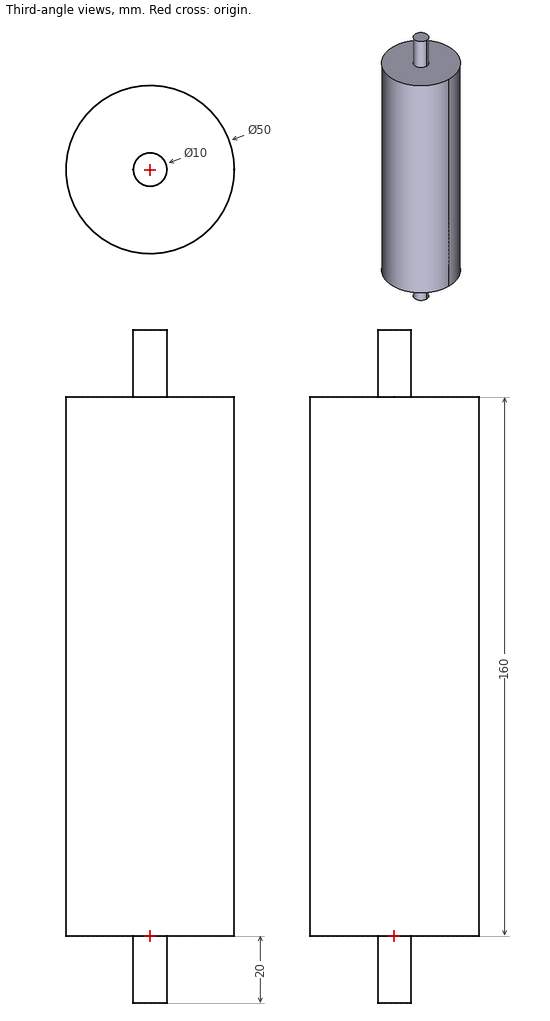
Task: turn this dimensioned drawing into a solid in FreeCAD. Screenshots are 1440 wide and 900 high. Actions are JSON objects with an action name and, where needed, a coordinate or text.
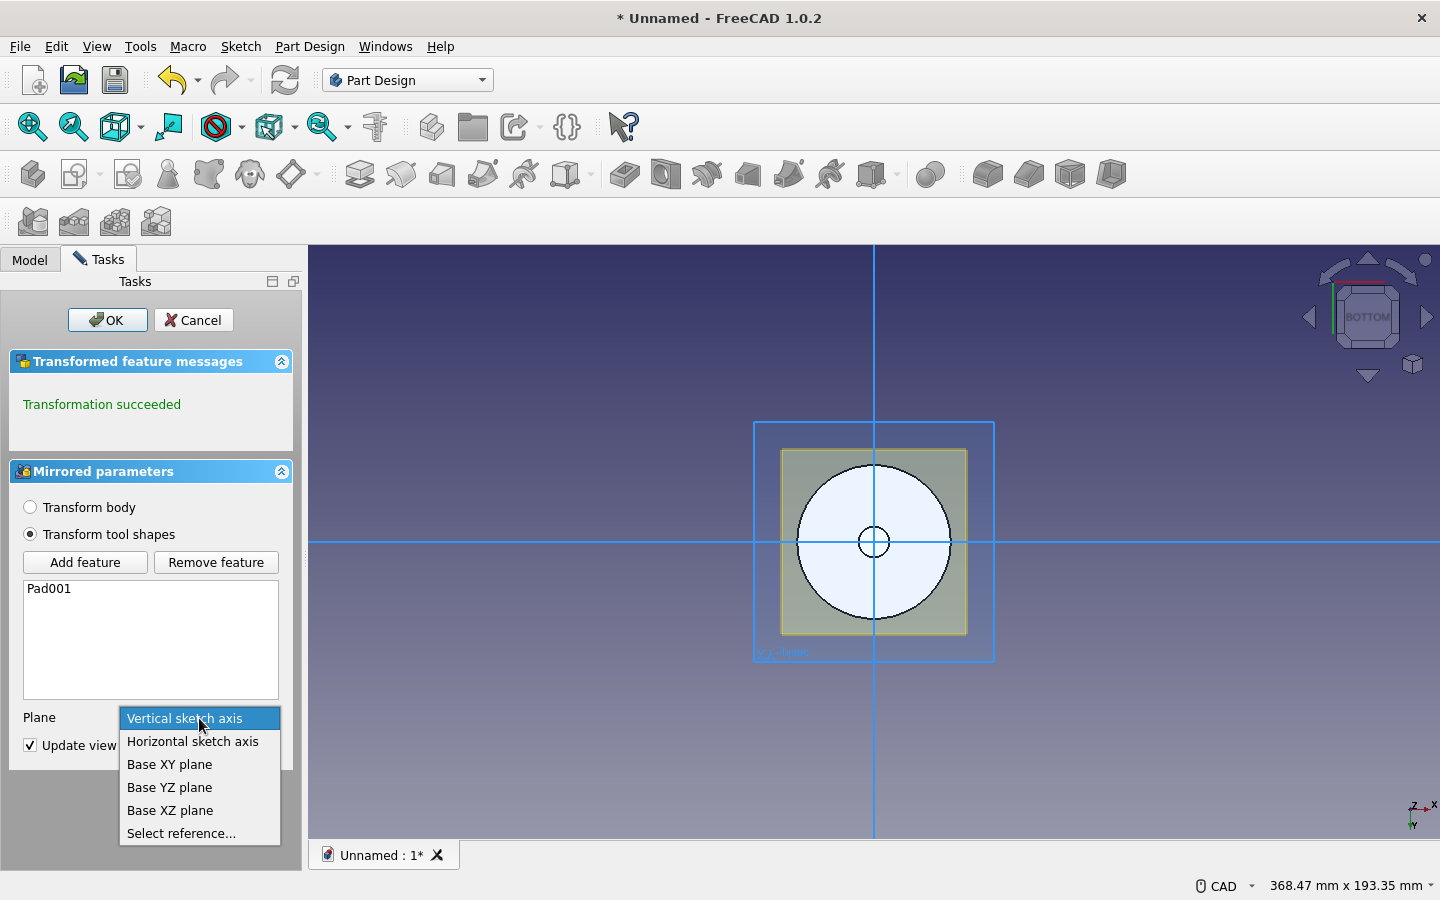
{"action": "left_click", "coordinate": [198, 834]}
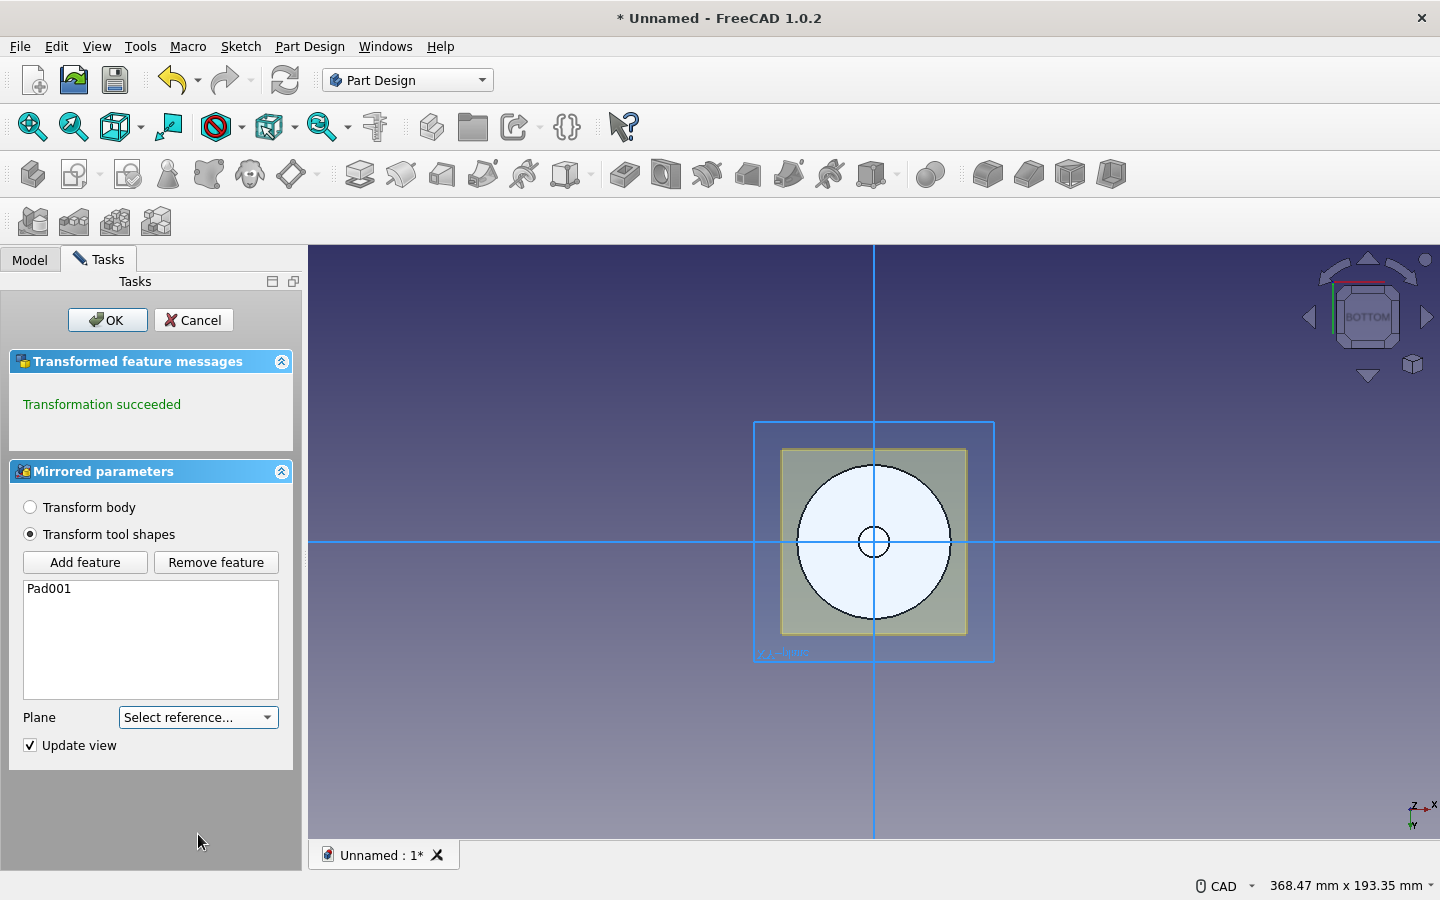
{"action": "left_click", "coordinate": [30, 259]}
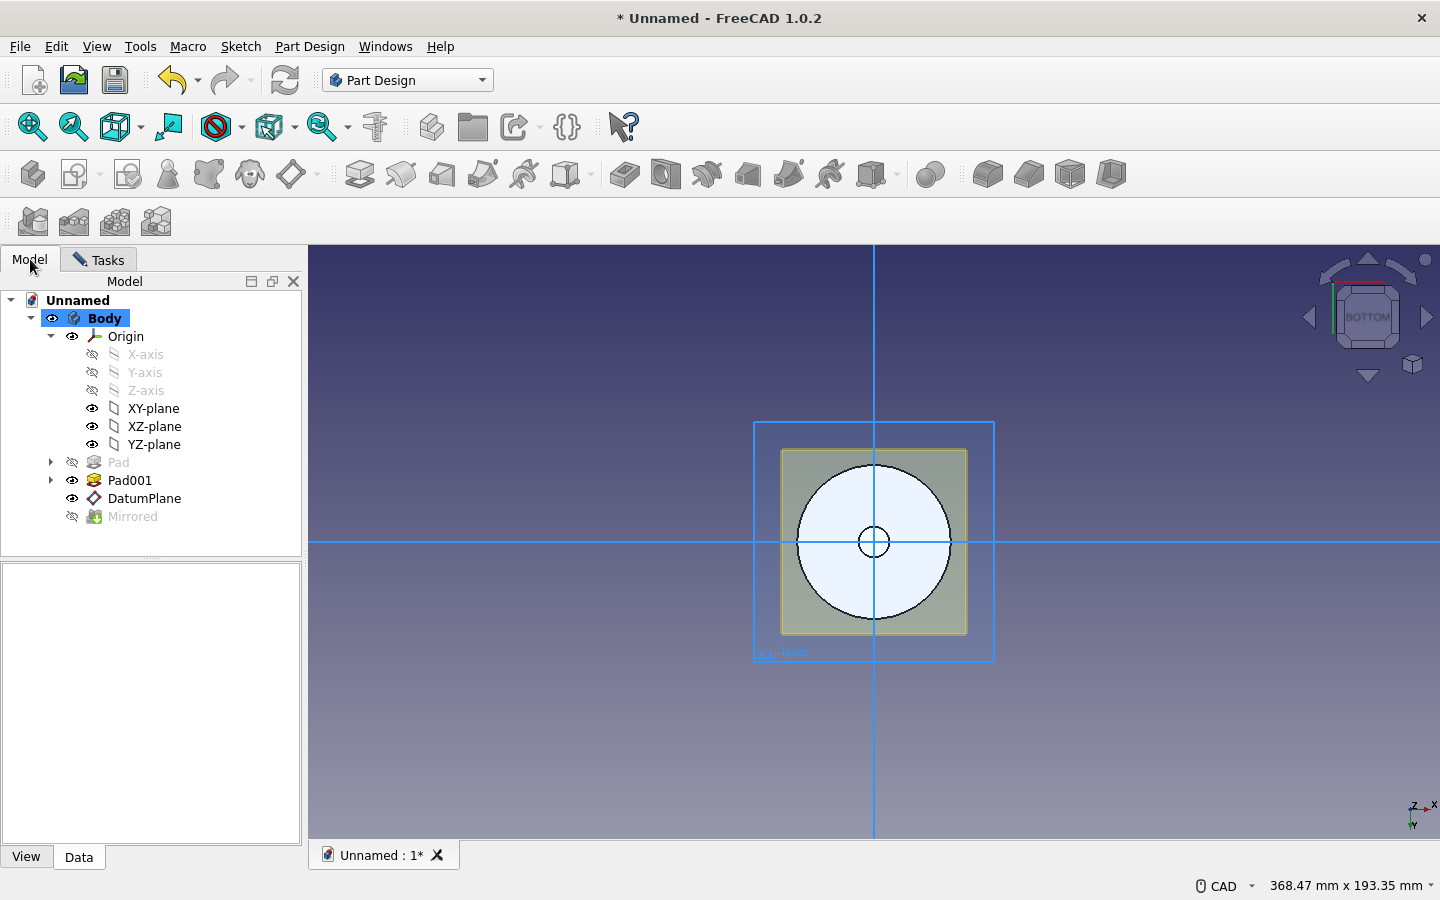
{"action": "left_click", "coordinate": [117, 498]}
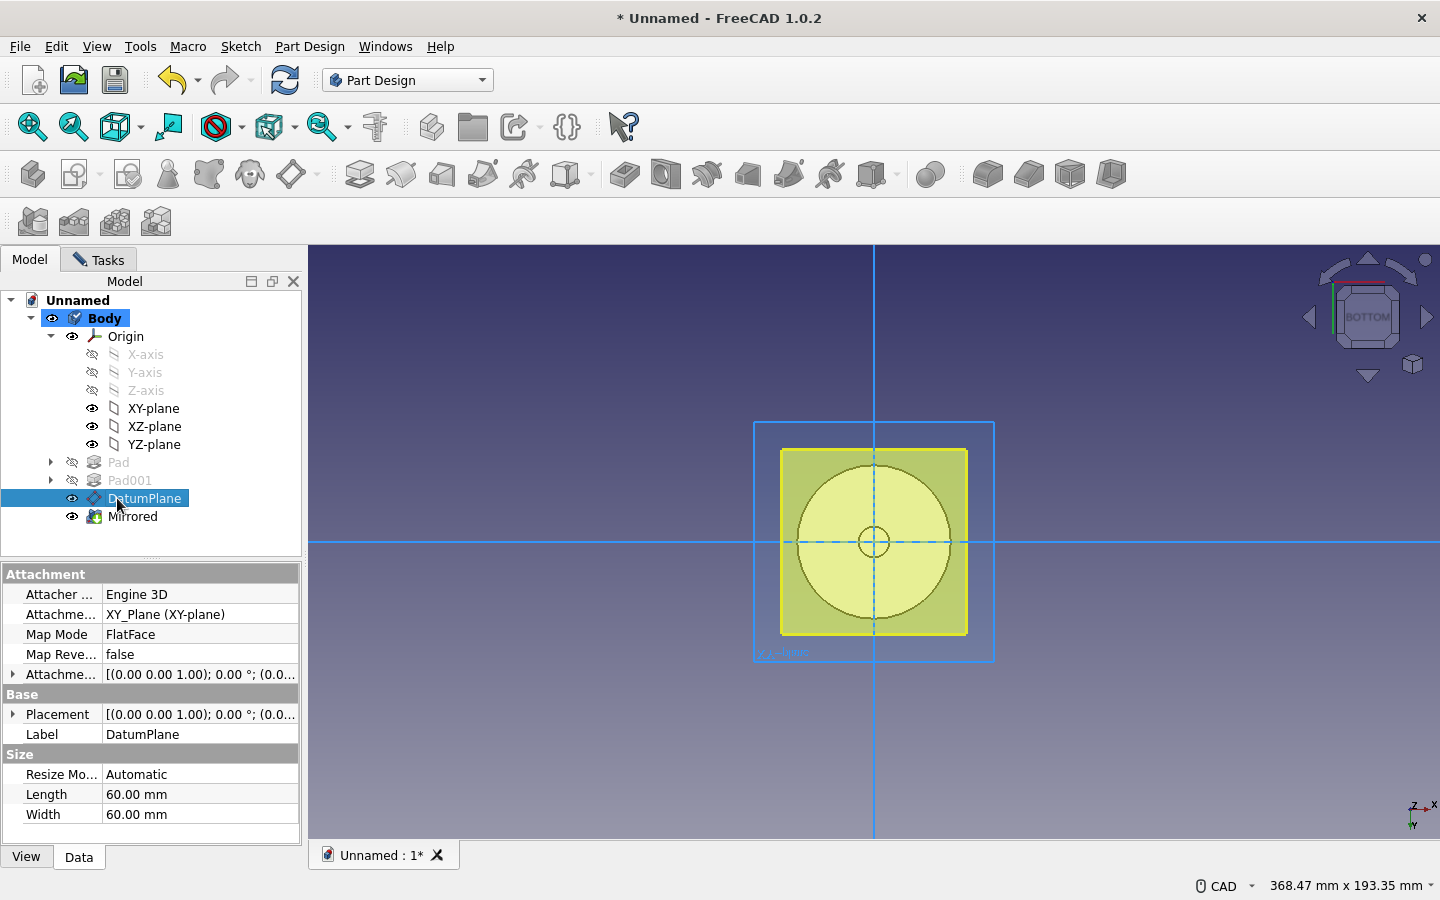
{"action": "left_click", "coordinate": [98, 259]}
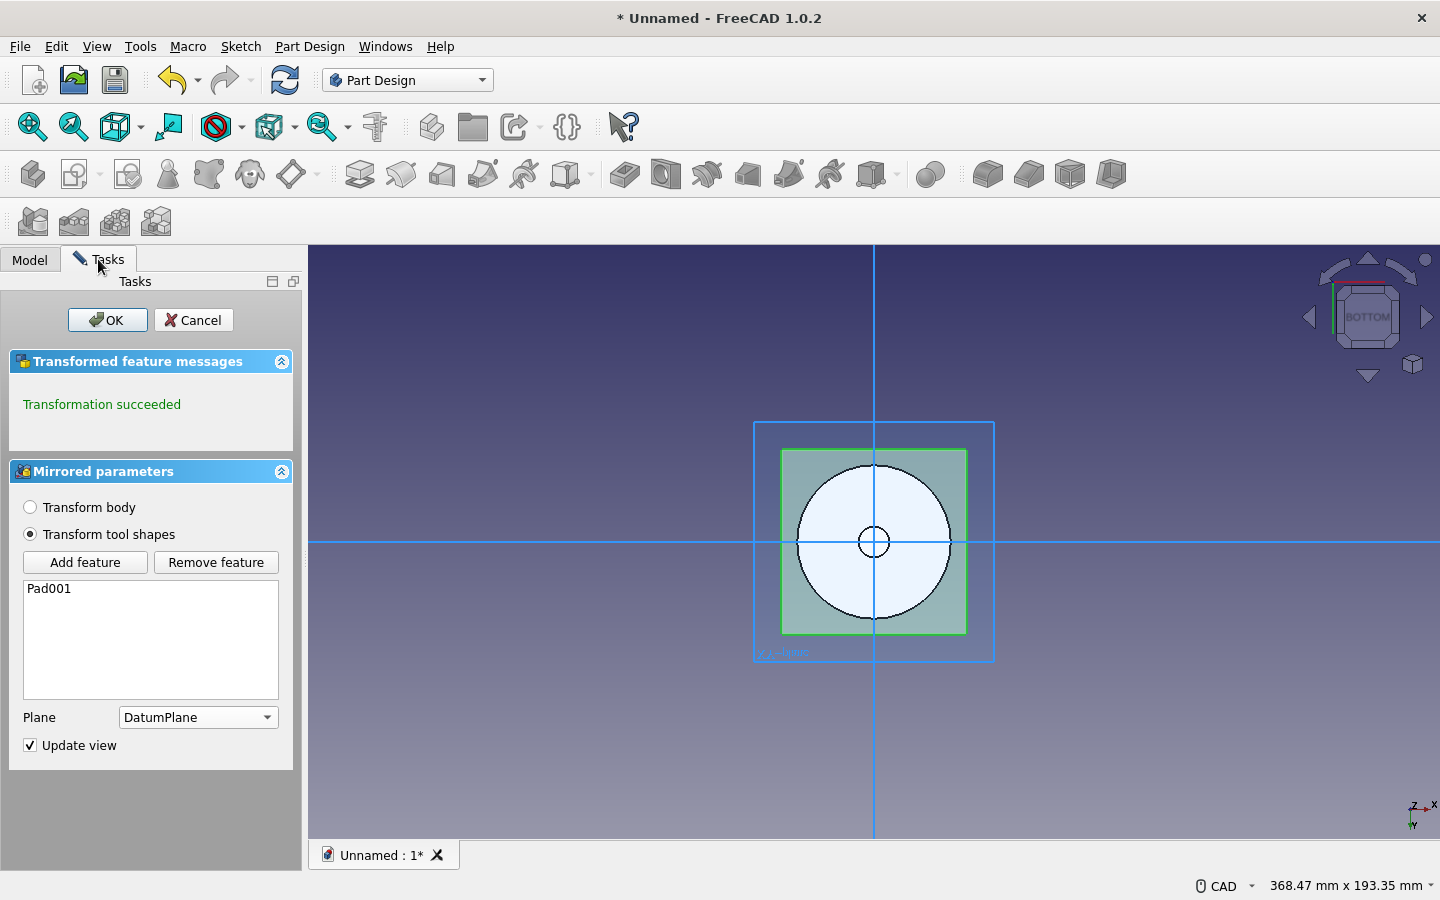
{"action": "left_click", "coordinate": [108, 320]}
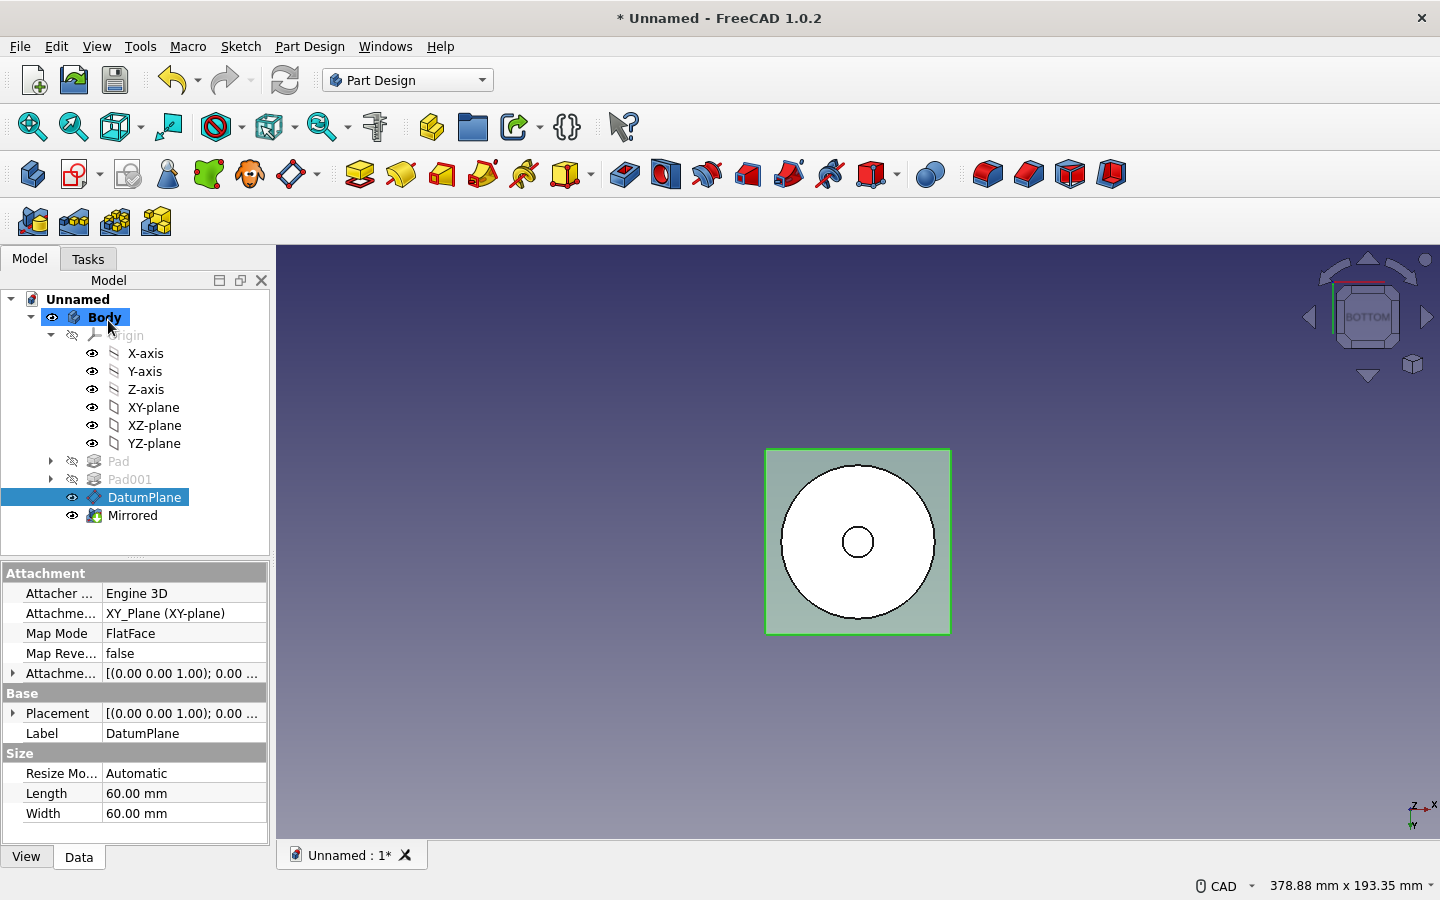
{"action": "left_click", "coordinate": [117, 497]}
{"action": "key", "text": "space"}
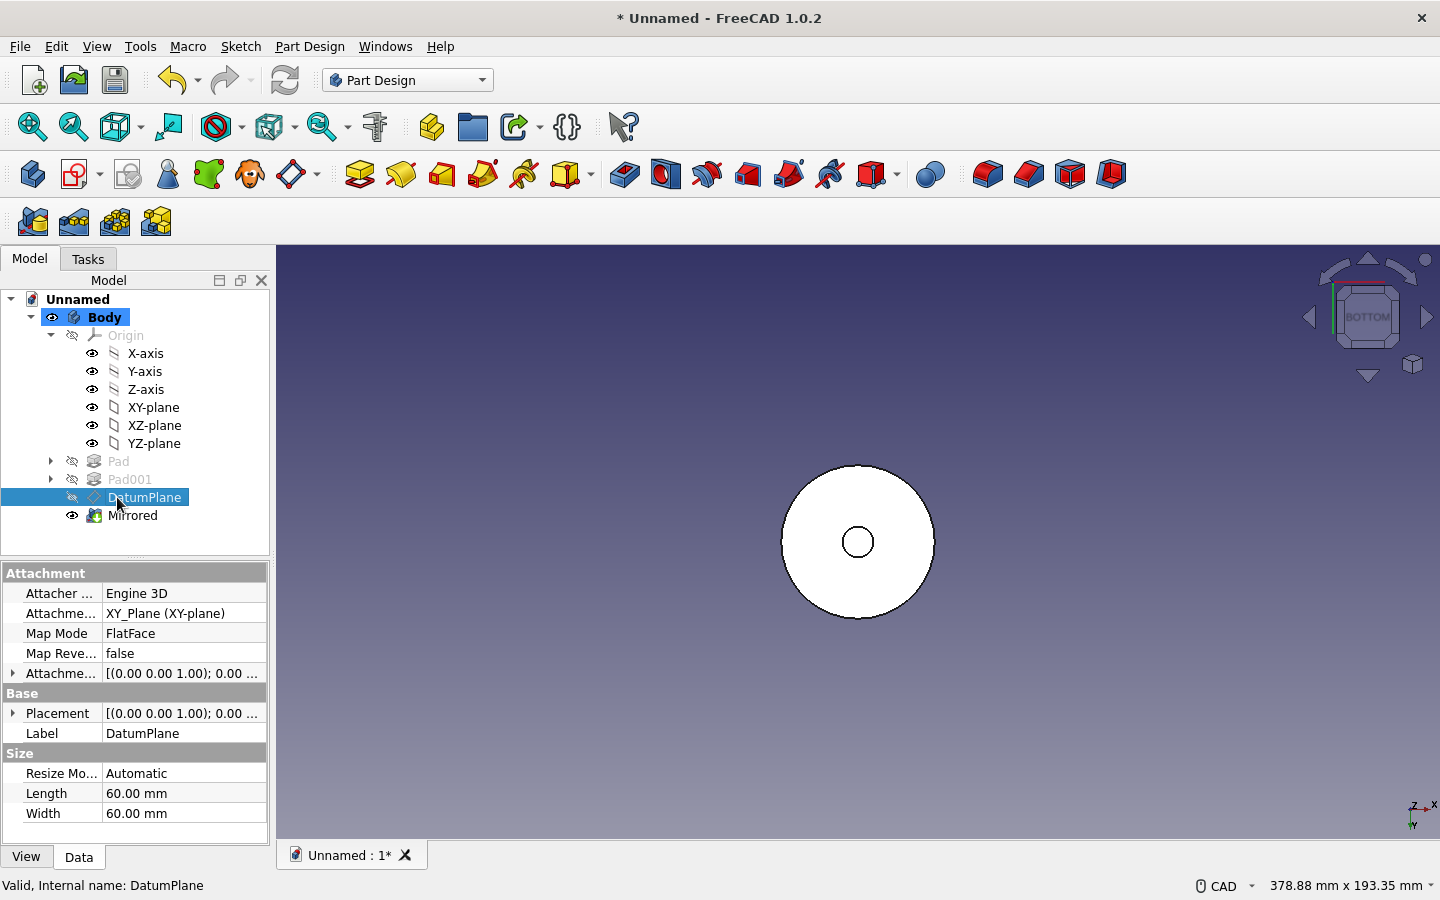
{"action": "key", "text": "0"}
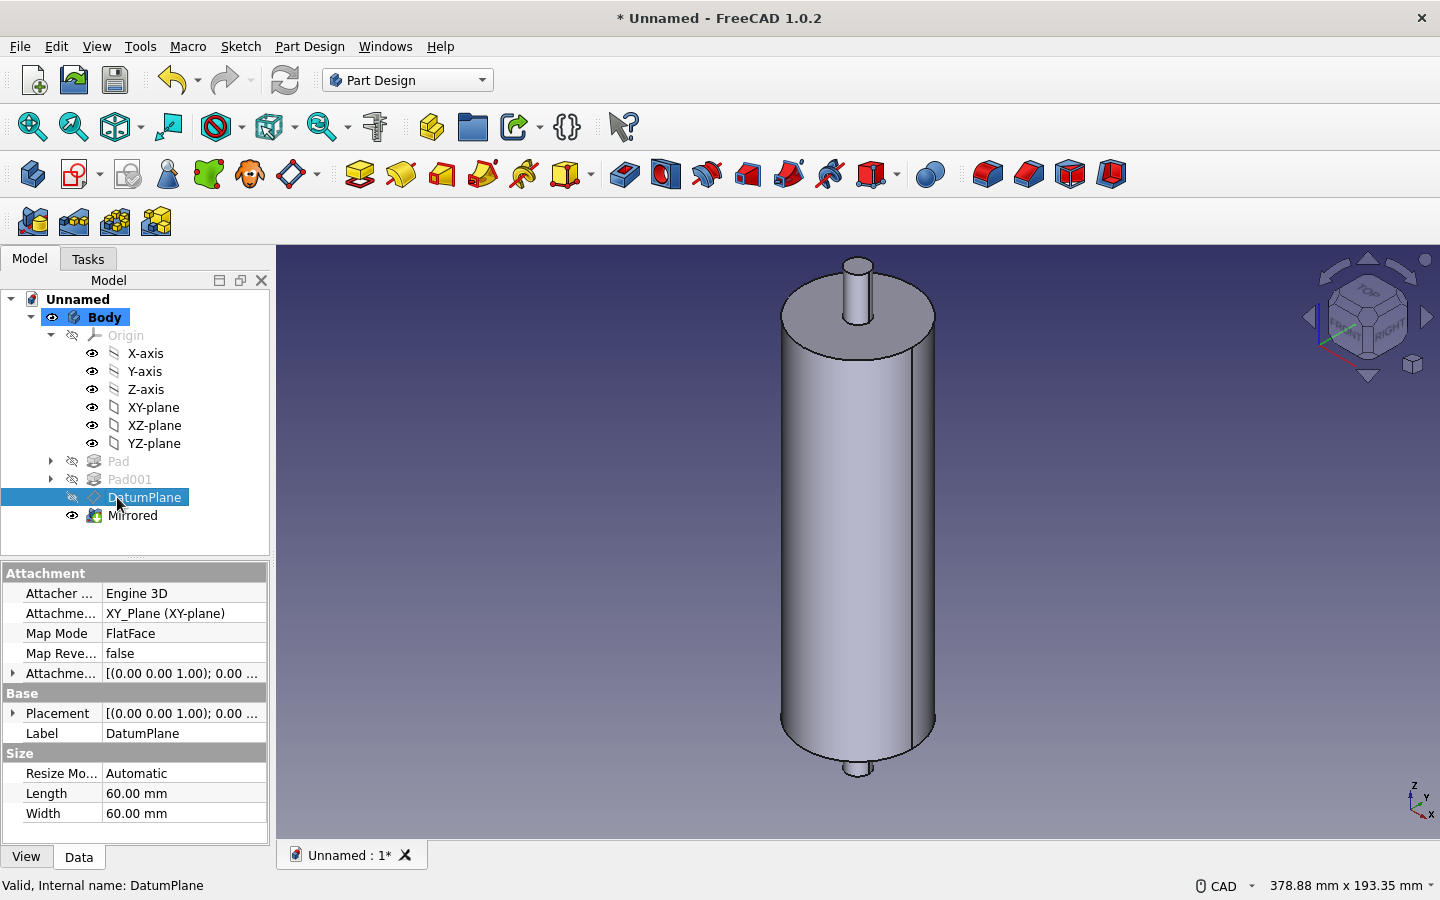
{"action": "left_click", "coordinate": [33, 128]}